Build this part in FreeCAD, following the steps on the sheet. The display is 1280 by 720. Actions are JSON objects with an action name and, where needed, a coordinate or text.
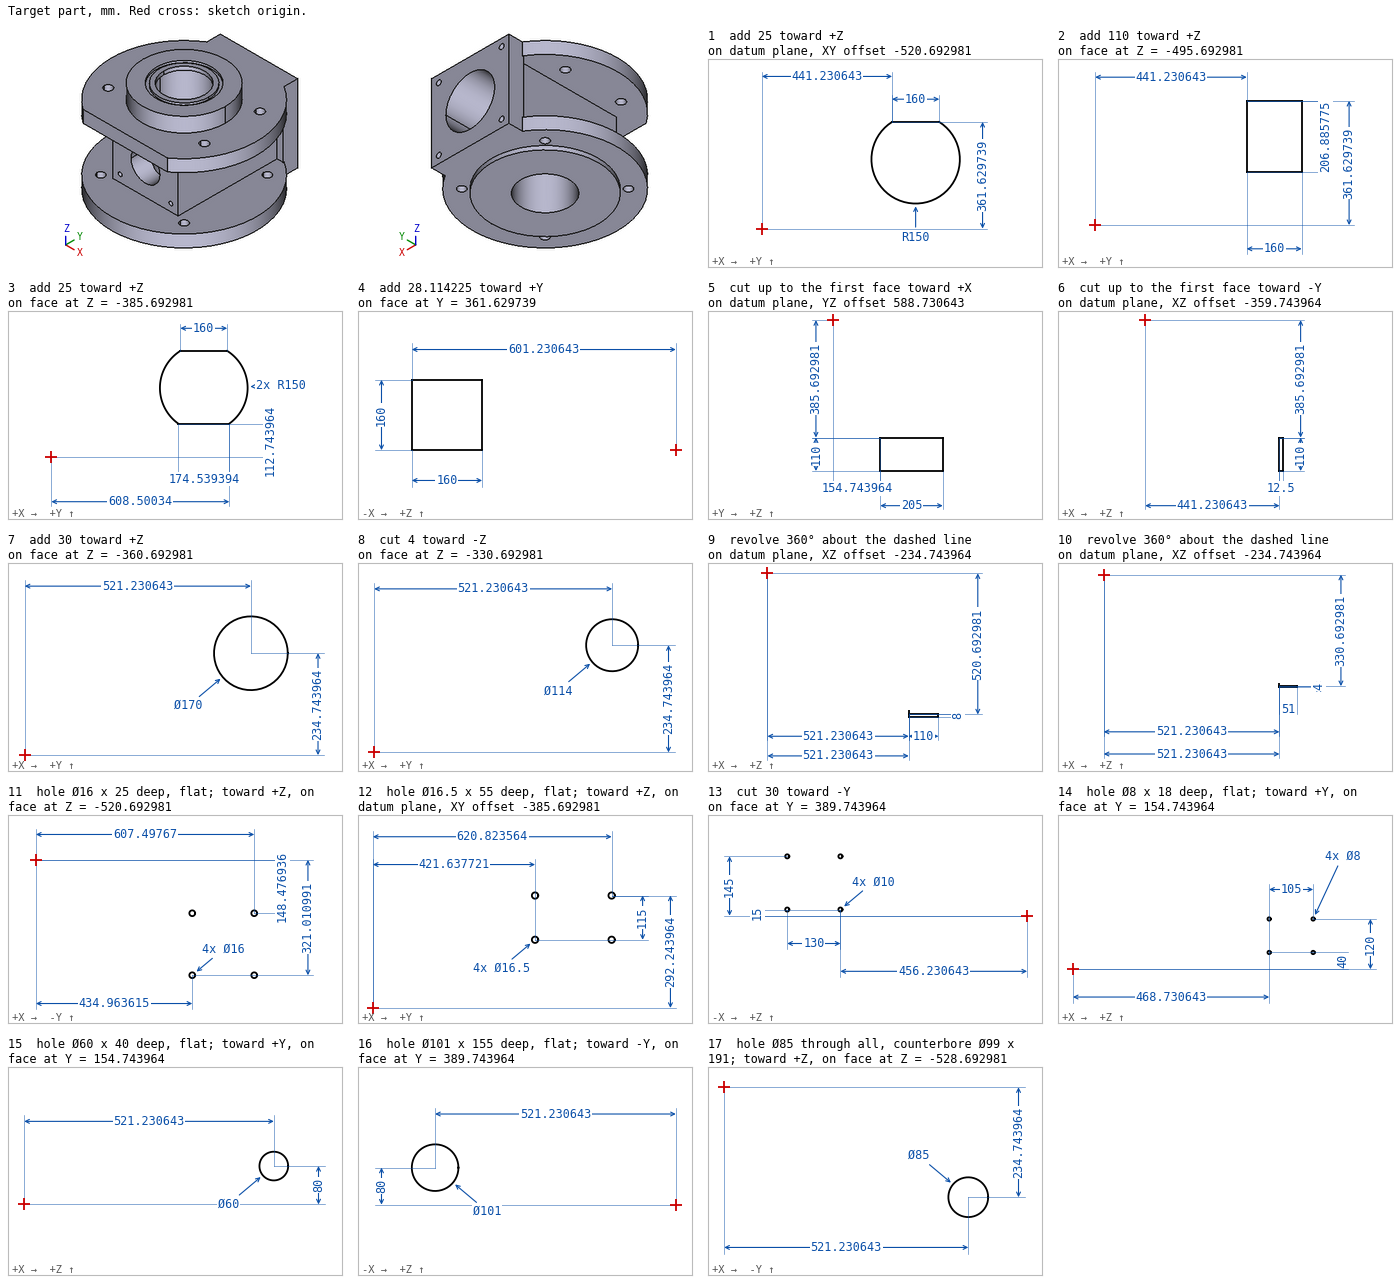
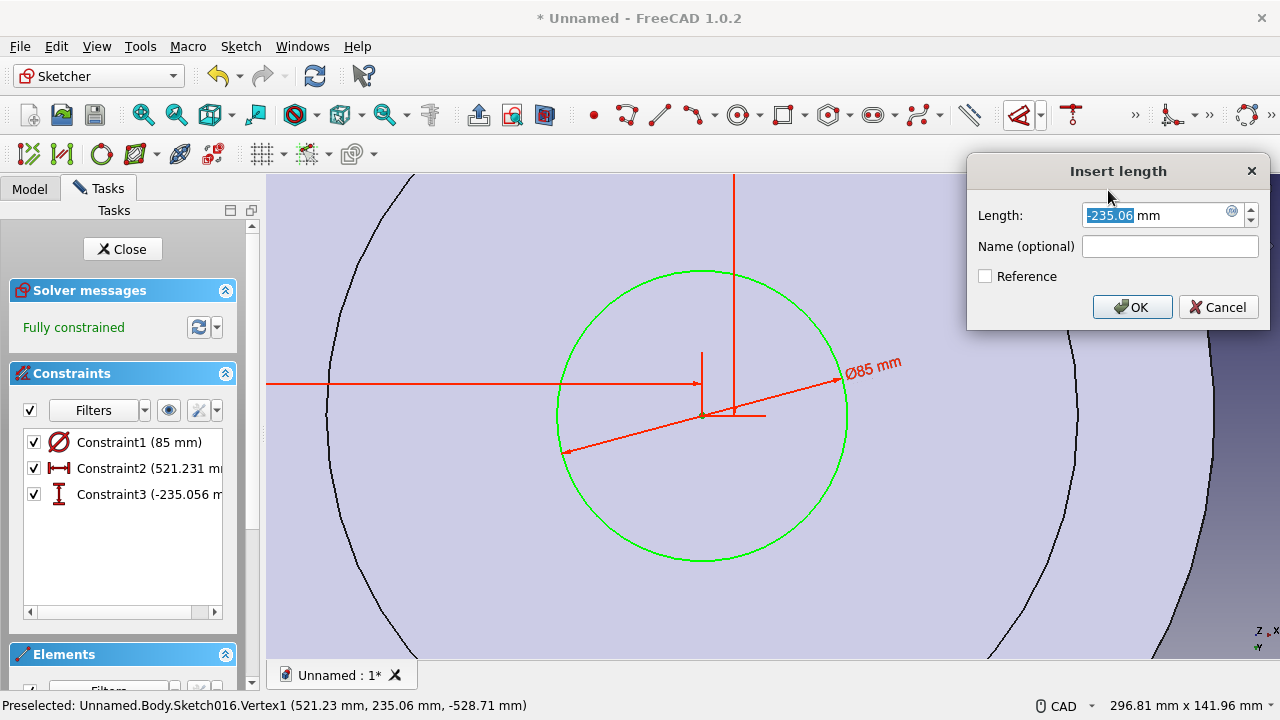
{"action": "type", "text": "-234.743964"}
{"action": "key", "text": "Return"}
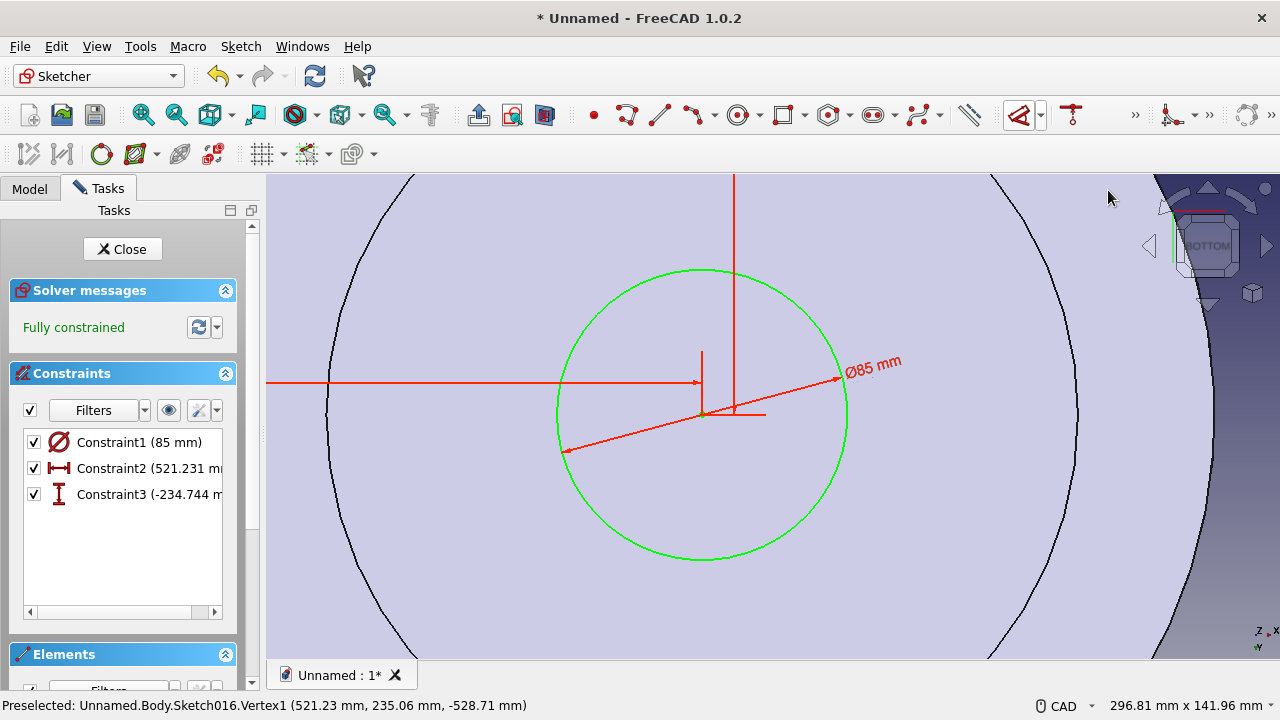
{"action": "left_click", "coordinate": [123, 249]}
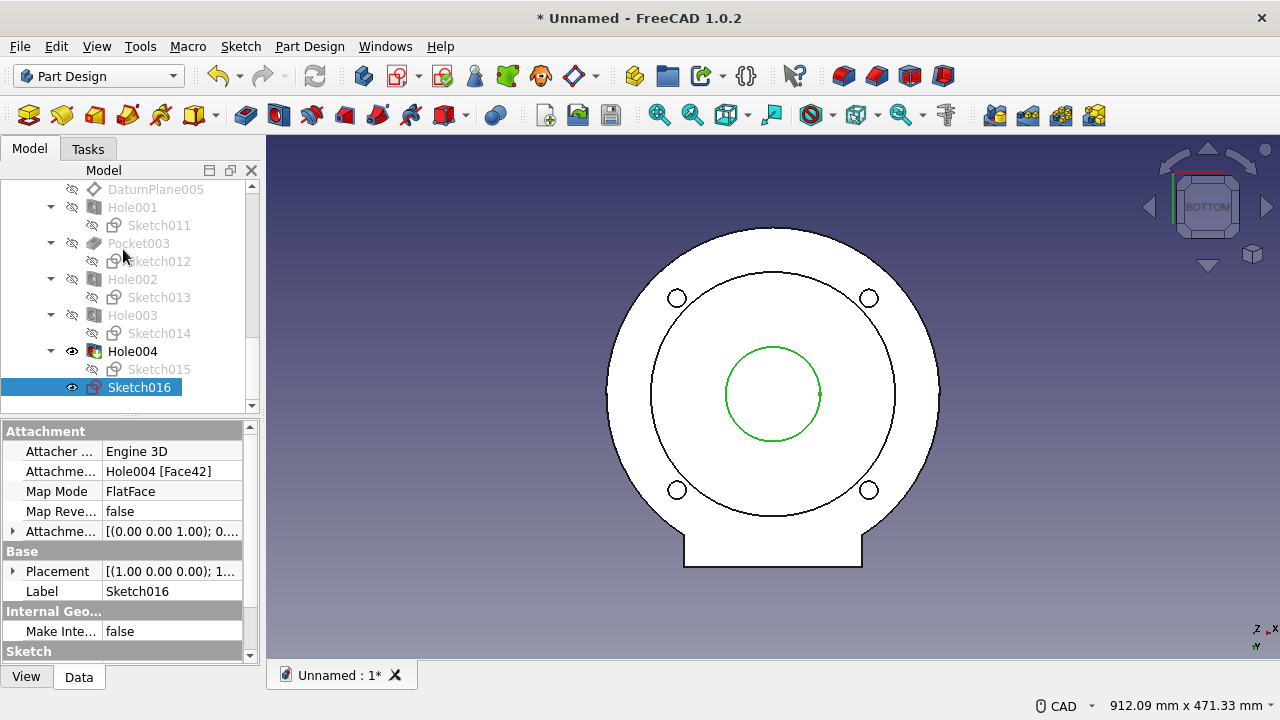
{"action": "left_click", "coordinate": [279, 116]}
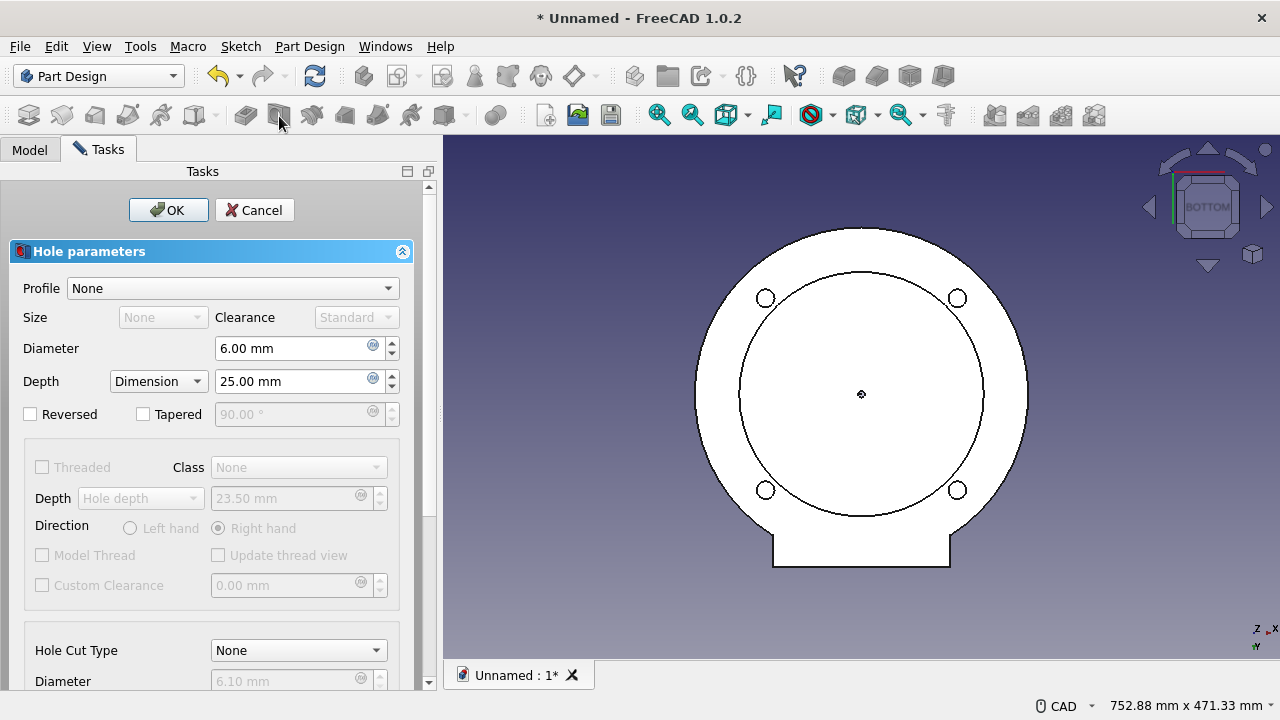
{"action": "triple_click", "coordinate": [300, 348]}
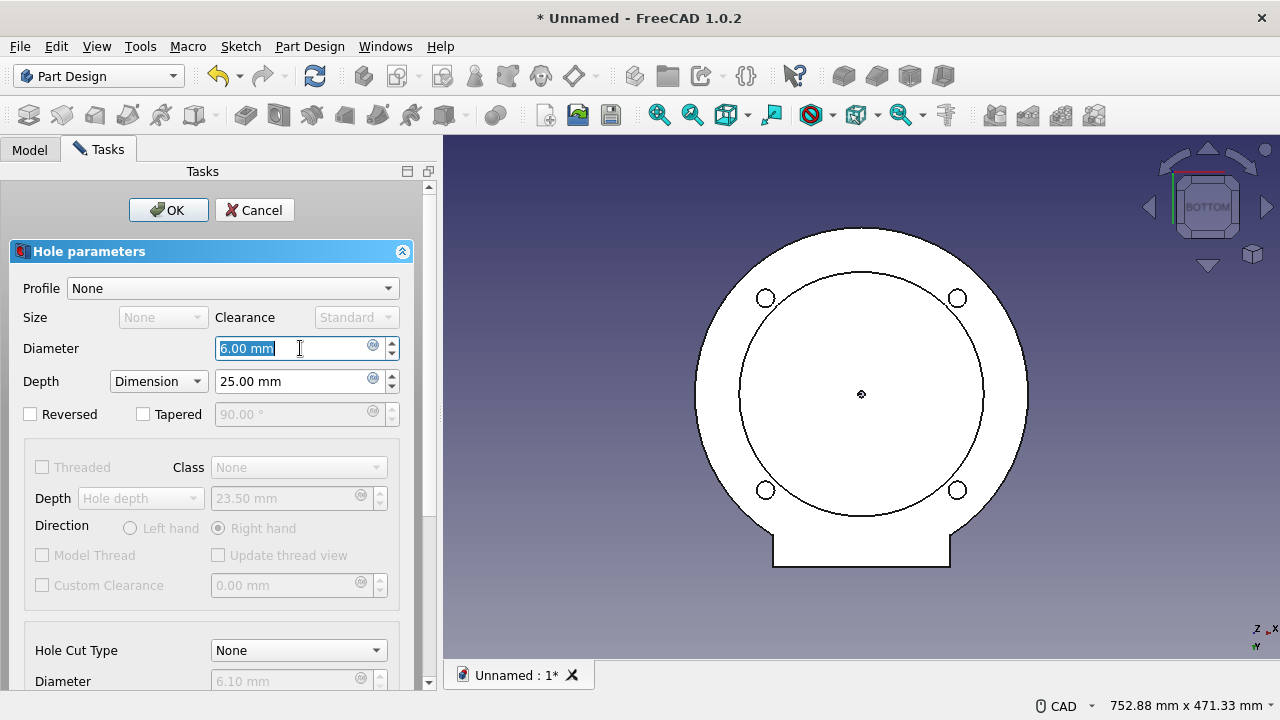
{"action": "type", "text": "85"}
{"action": "key", "text": "Tab"}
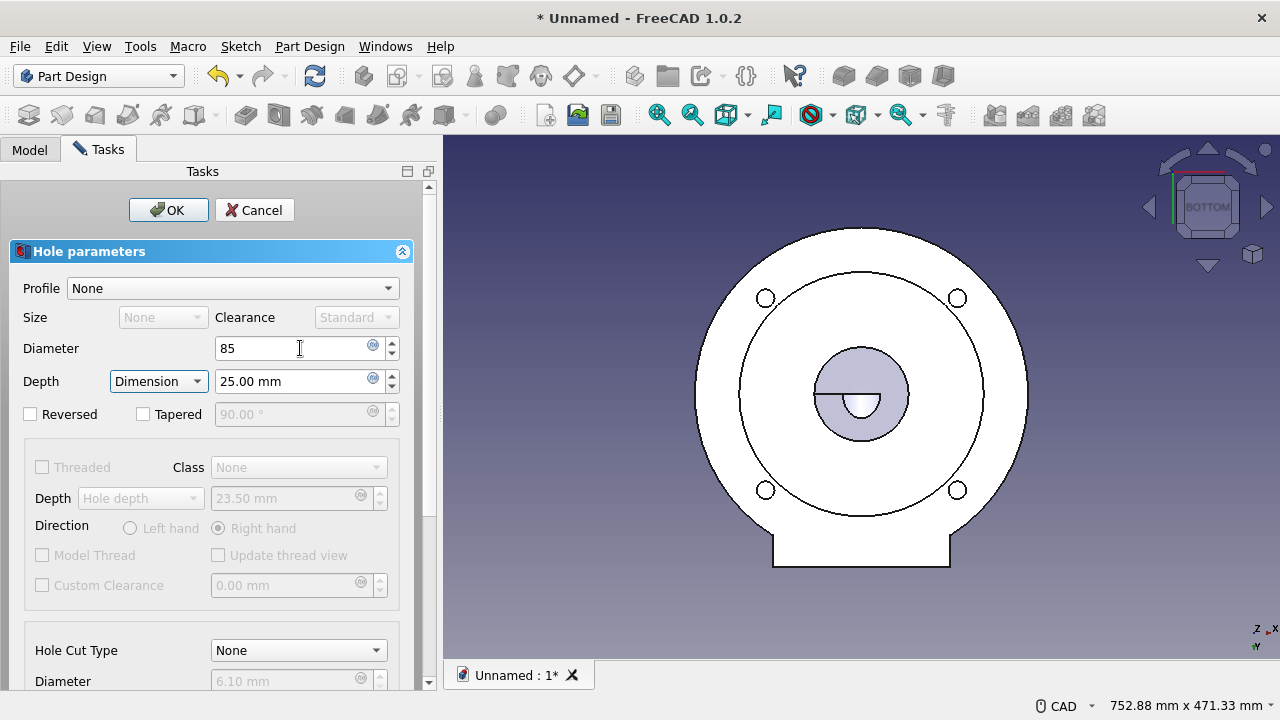
{"action": "left_click", "coordinate": [160, 382]}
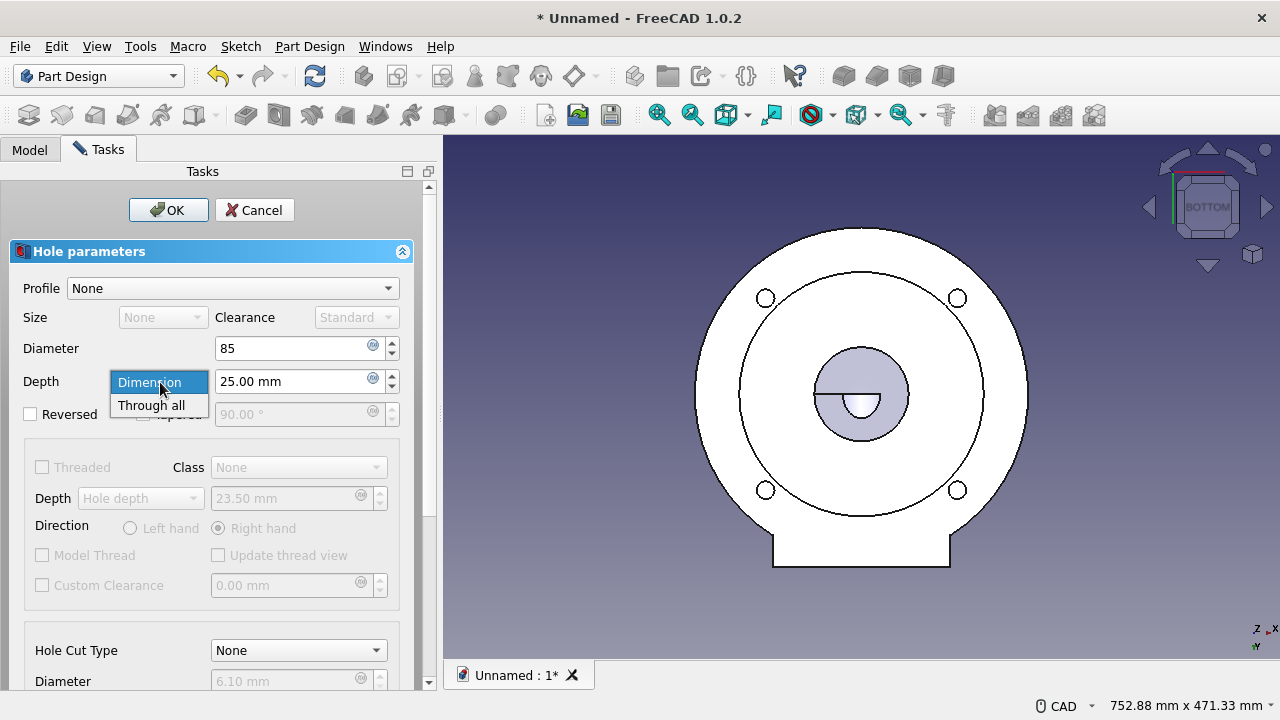
{"action": "left_click", "coordinate": [158, 406]}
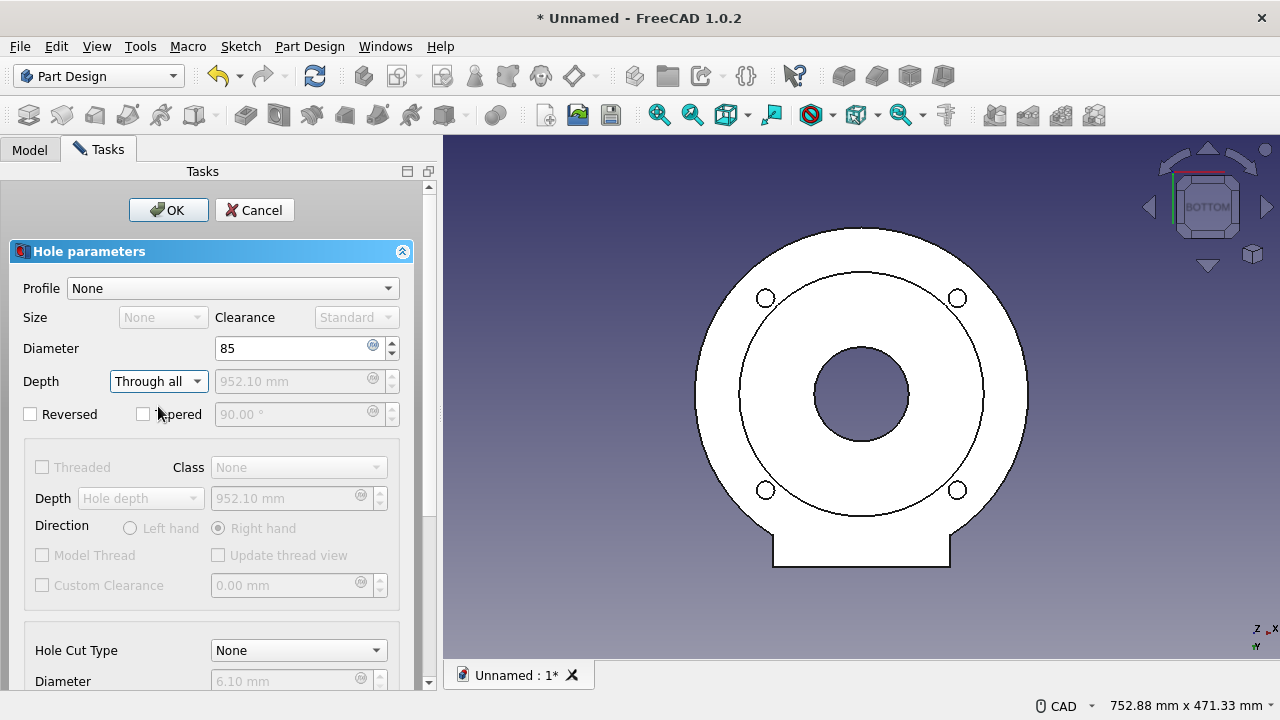
{"action": "left_click", "coordinate": [300, 650]}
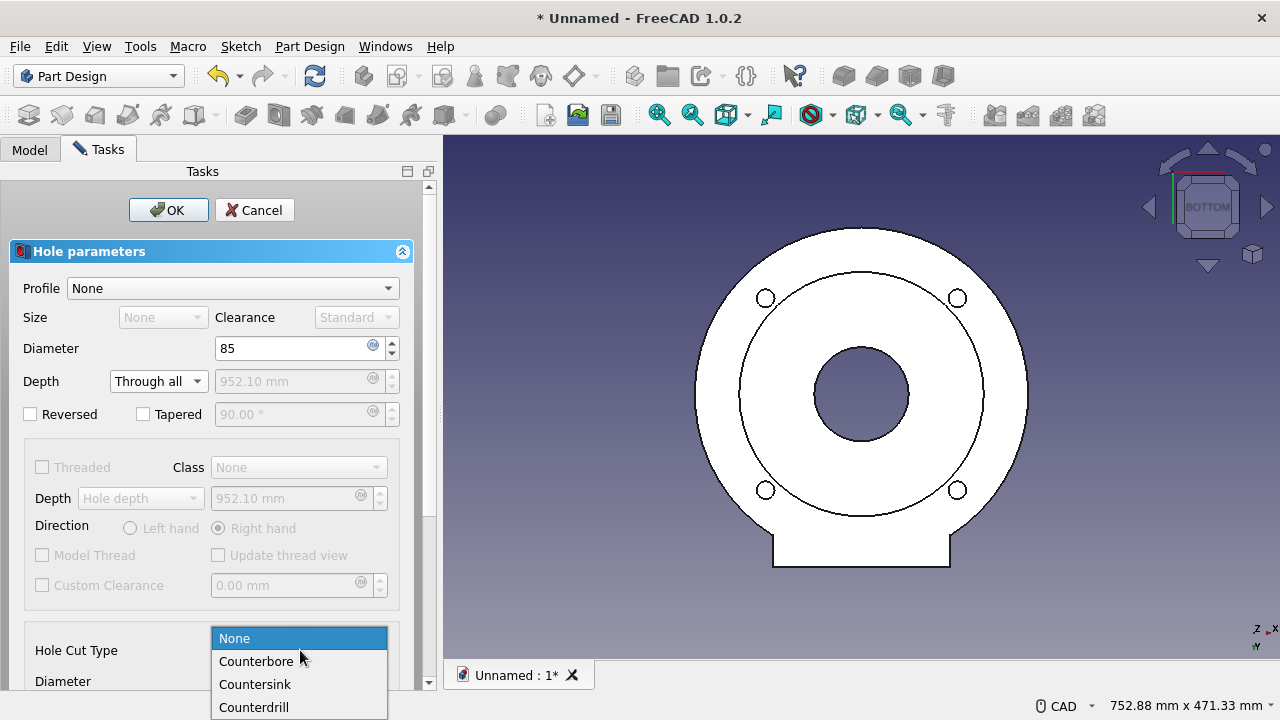
{"action": "left_click", "coordinate": [298, 662]}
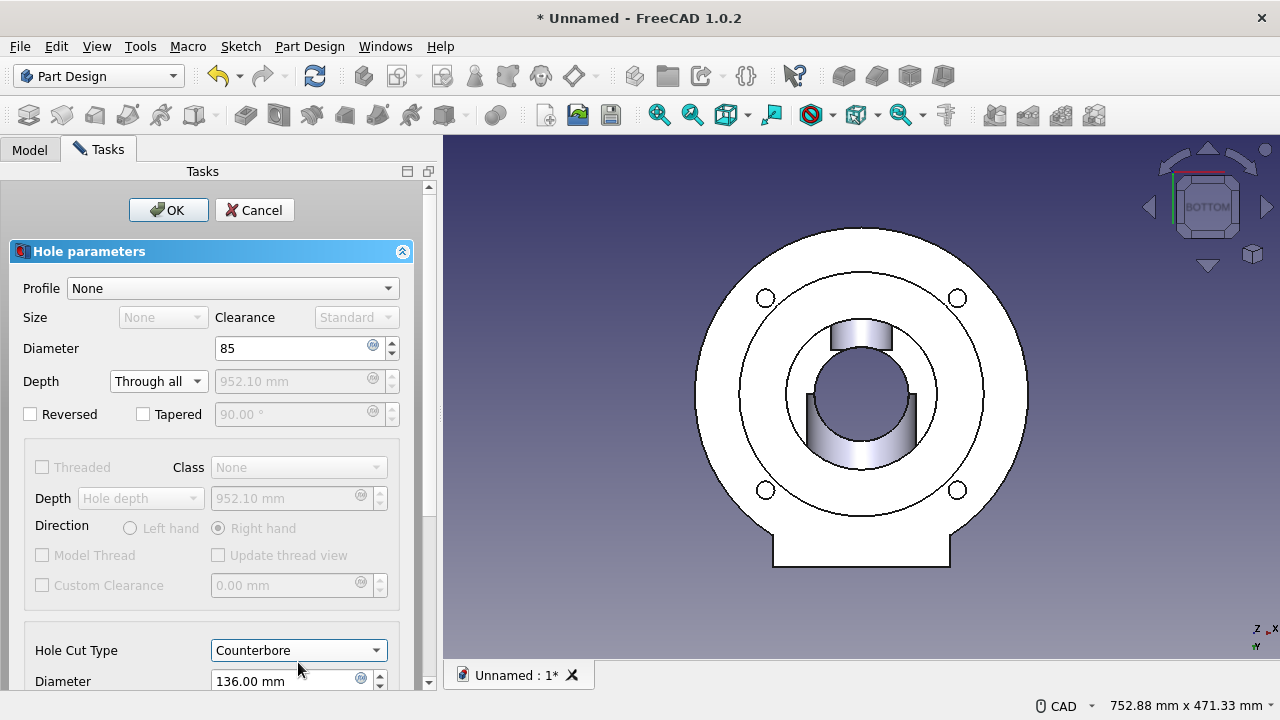
{"action": "scroll", "coordinate": [429, 436], "scroll_direction": "down", "scroll_amount": 2}